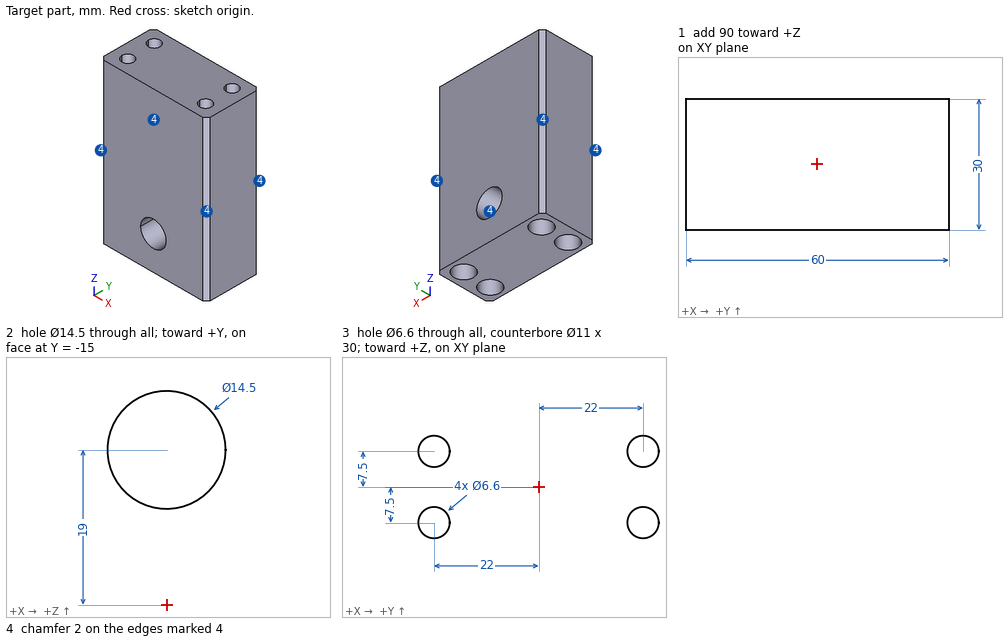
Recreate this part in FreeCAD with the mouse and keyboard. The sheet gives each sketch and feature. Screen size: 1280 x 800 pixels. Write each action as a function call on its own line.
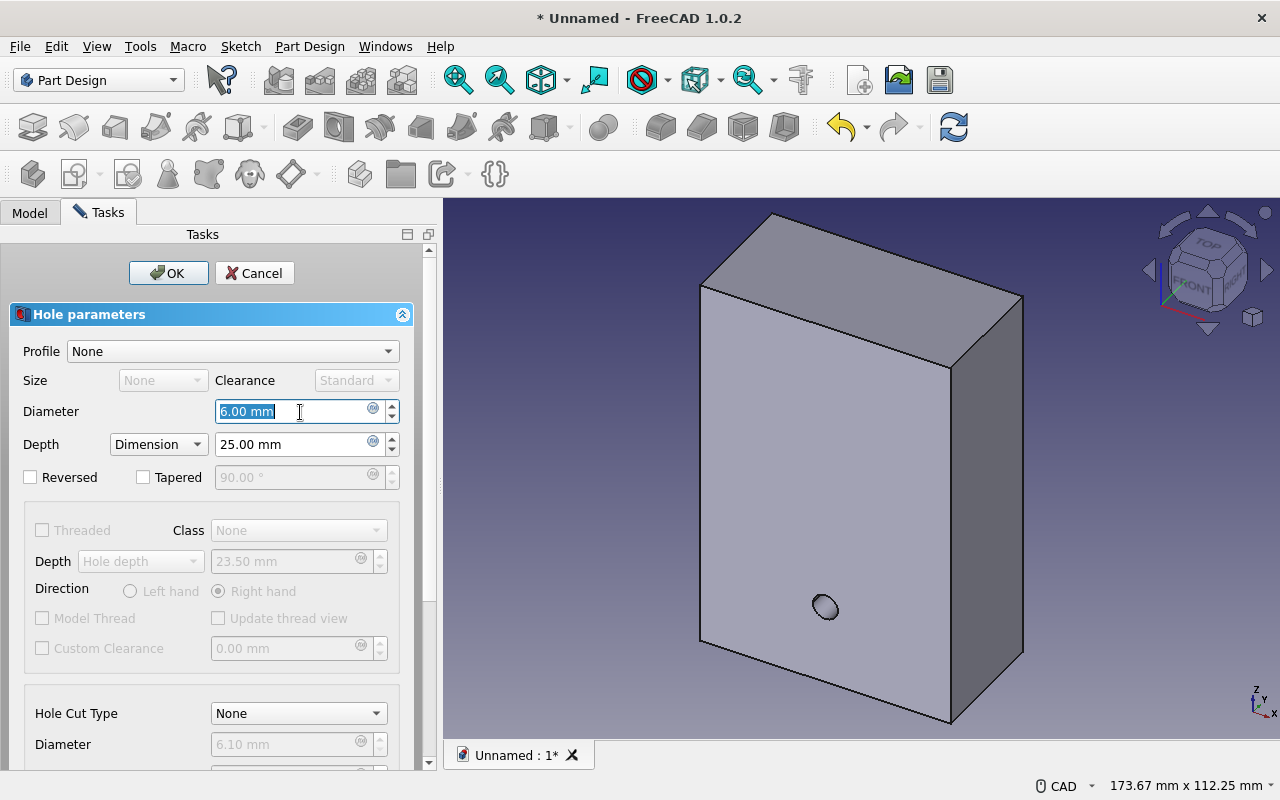
text(14.5)
key(Tab)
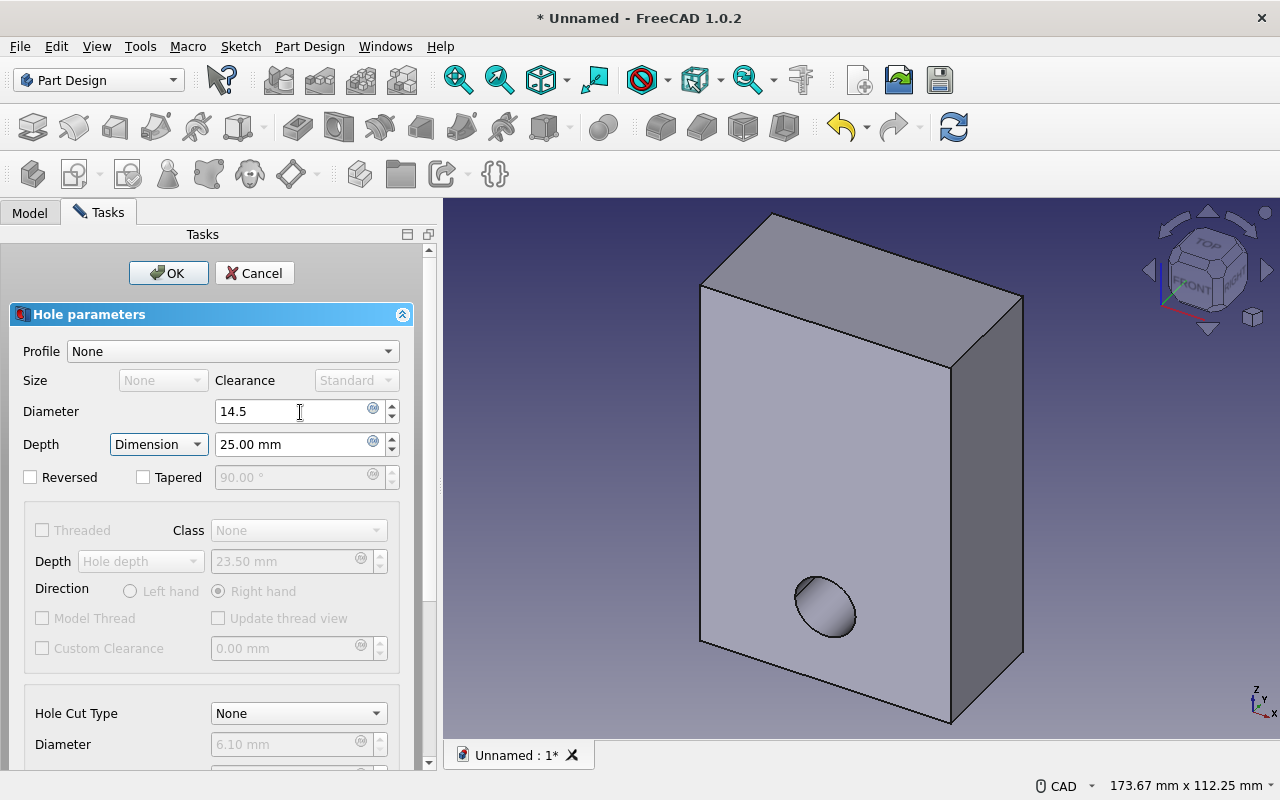
click(160, 444)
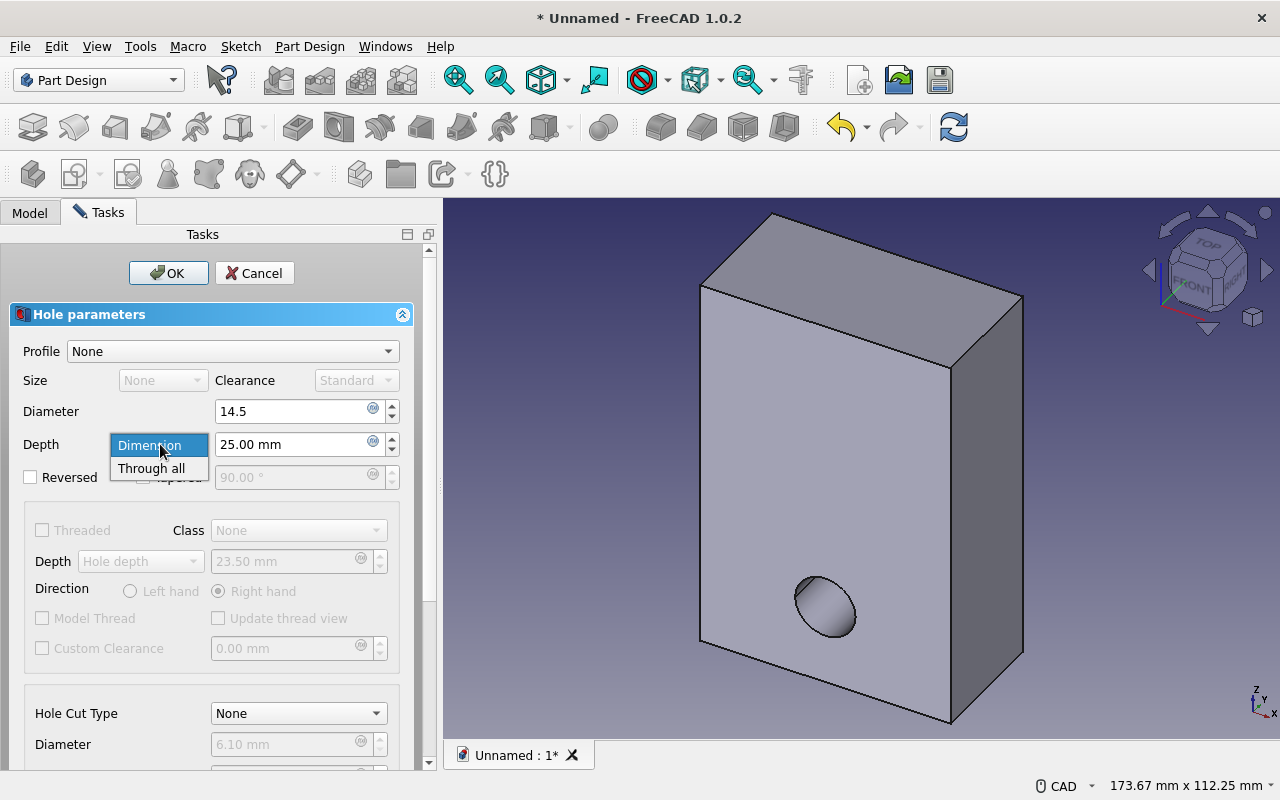
click(158, 468)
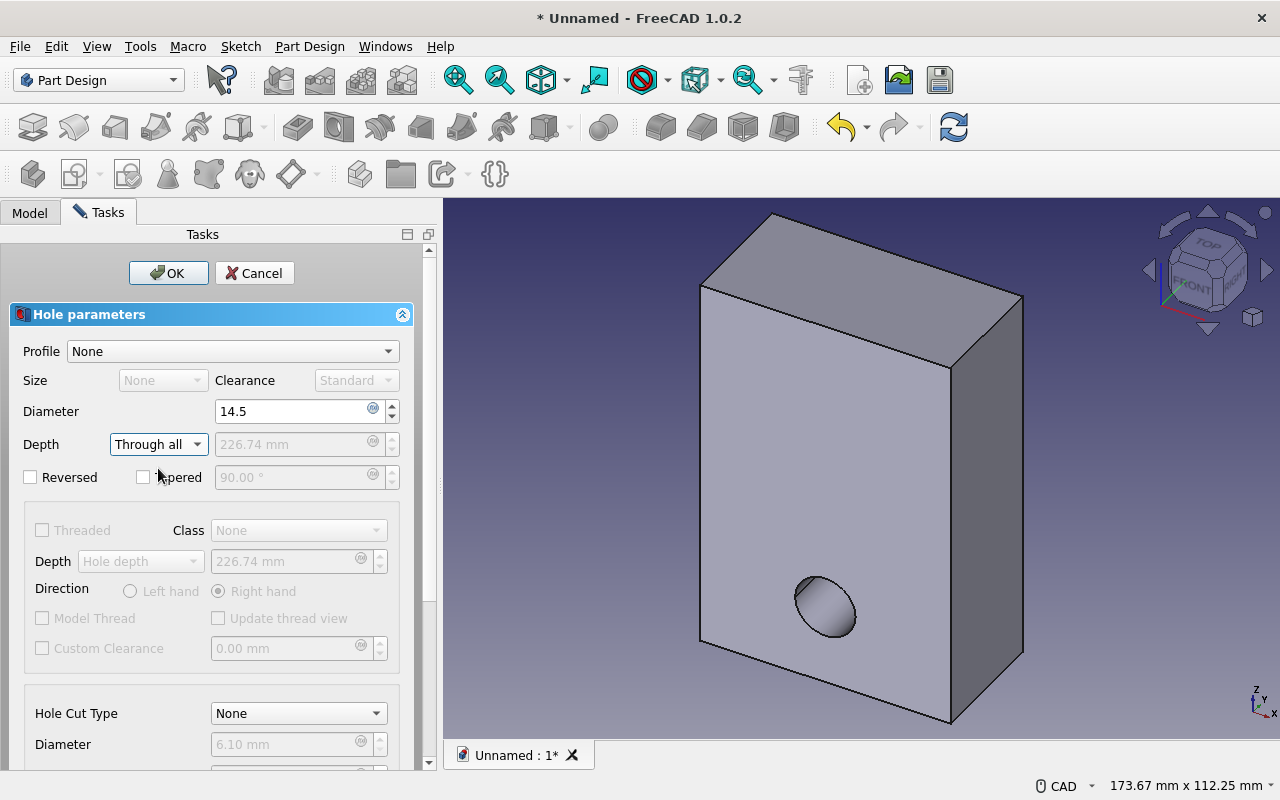
click(169, 273)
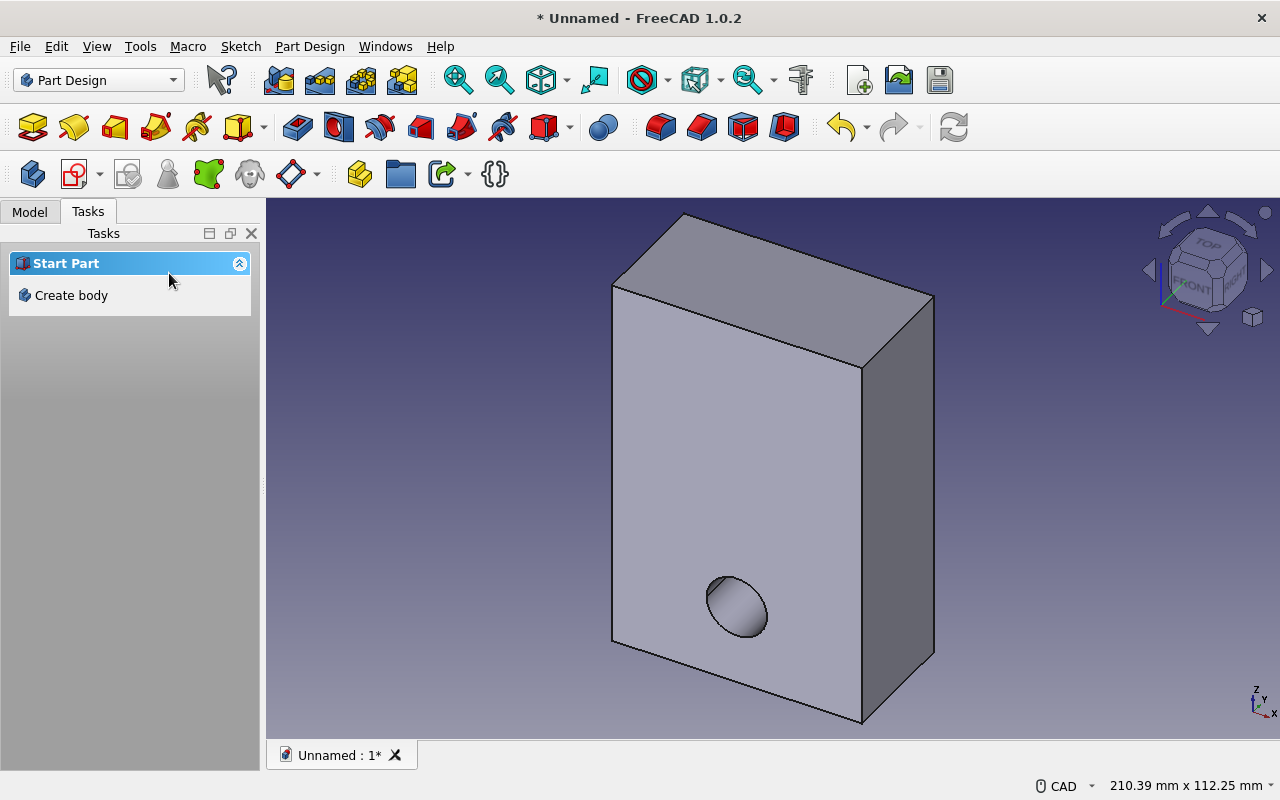
click(74, 174)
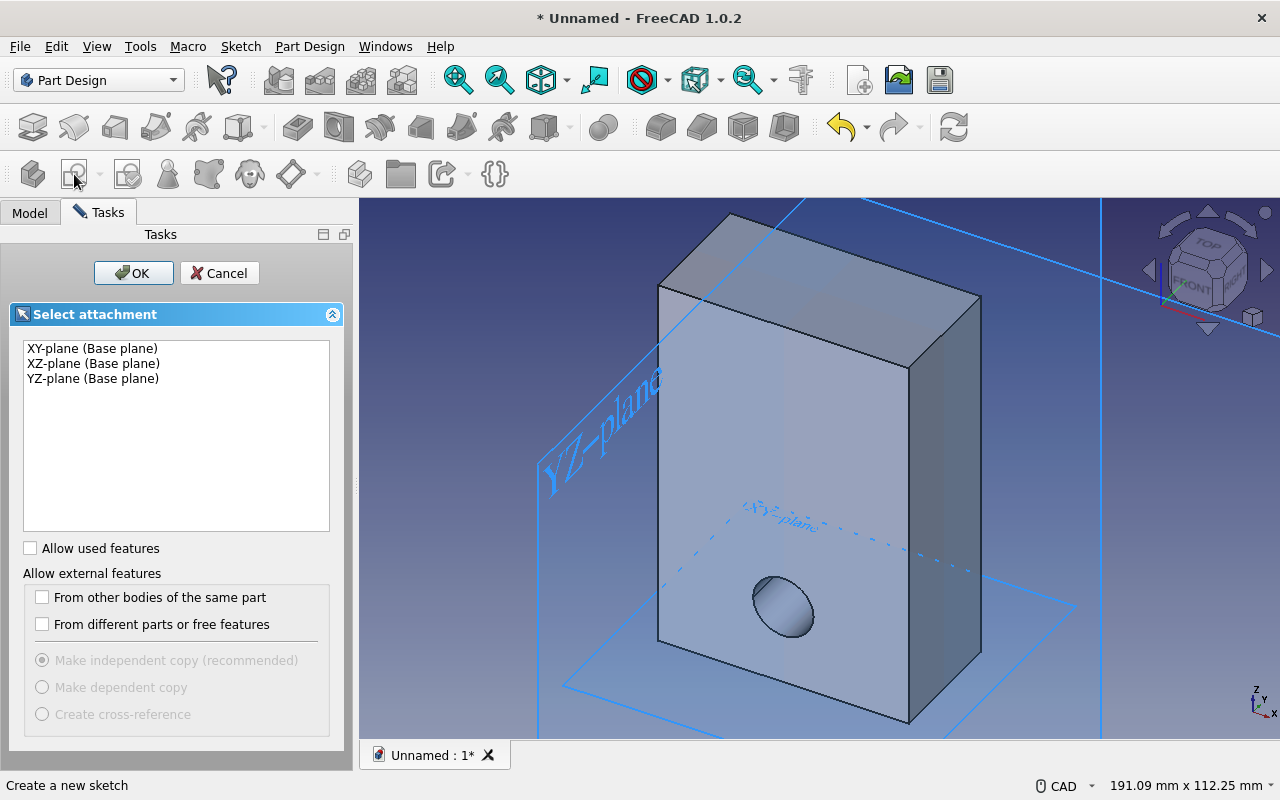
click(84, 348)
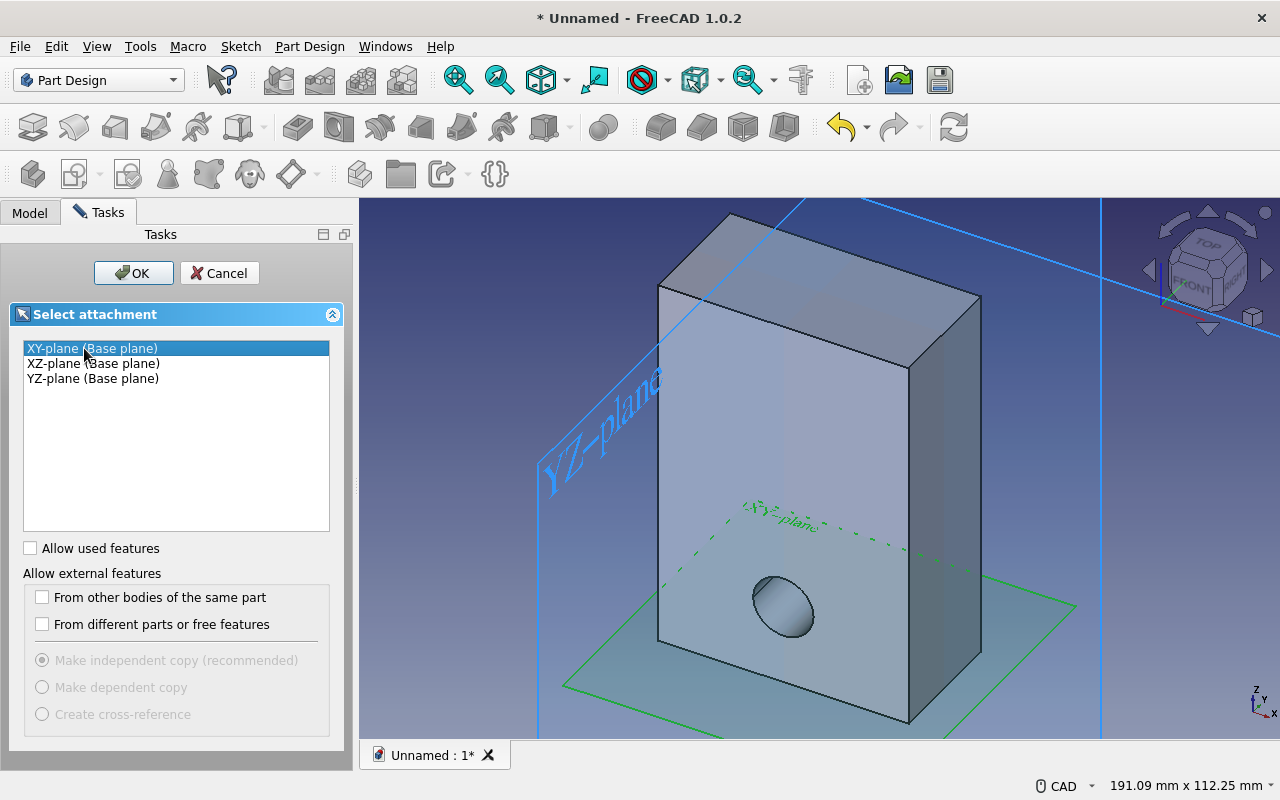
click(134, 273)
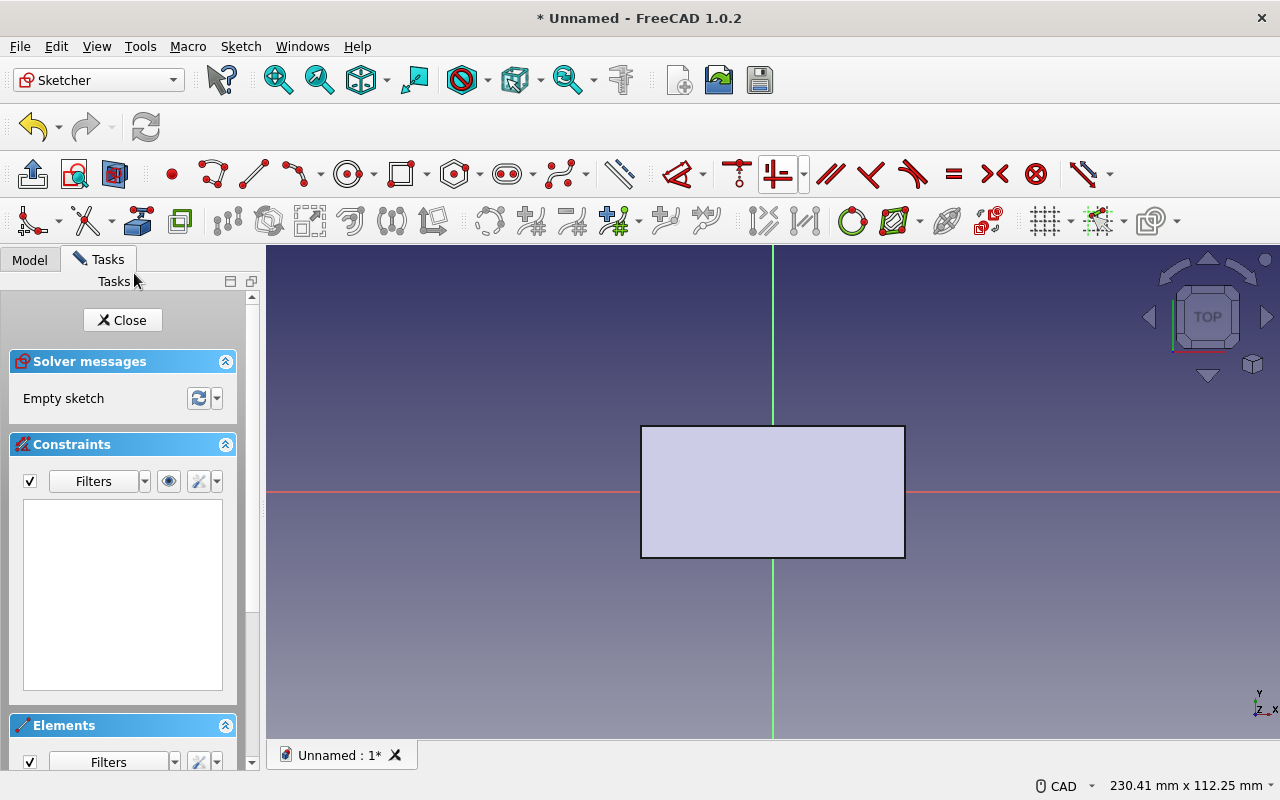
click(115, 174)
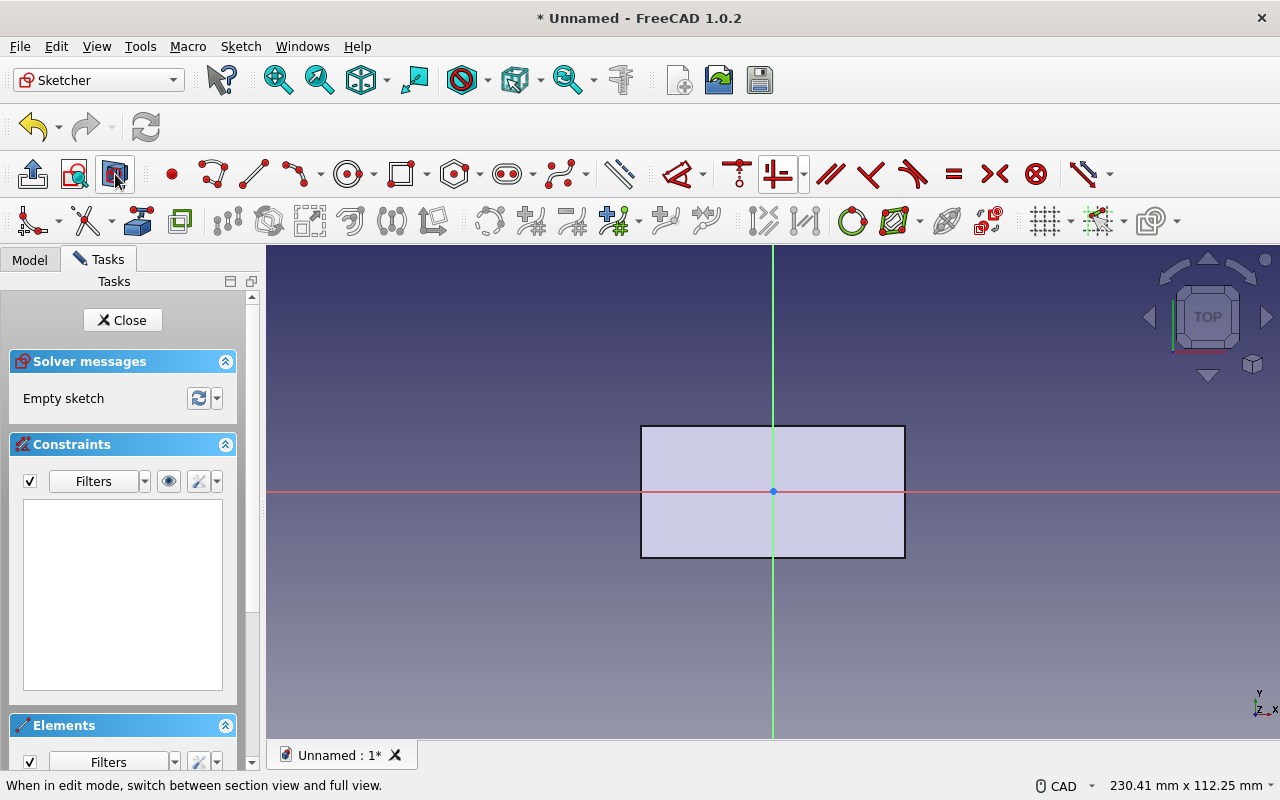
scroll(813, 492, up, 5)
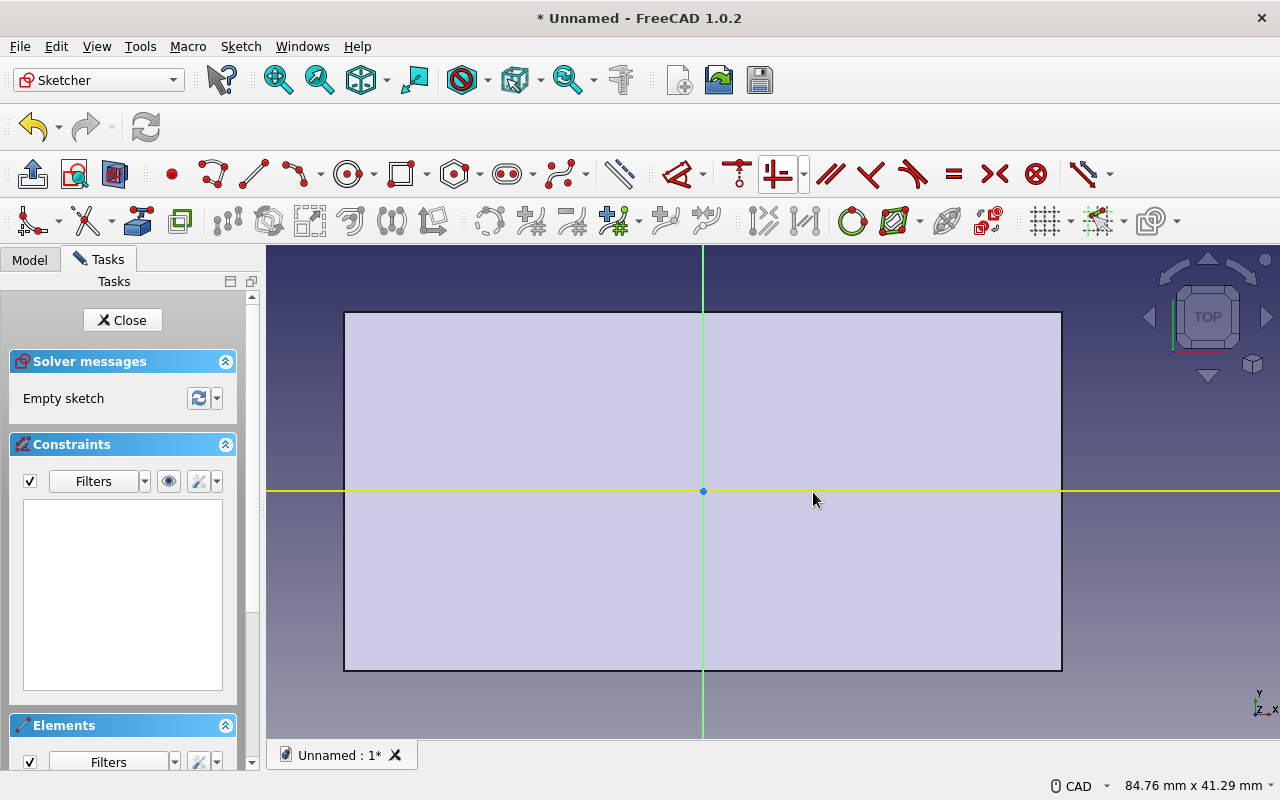
key(g)
key(c)